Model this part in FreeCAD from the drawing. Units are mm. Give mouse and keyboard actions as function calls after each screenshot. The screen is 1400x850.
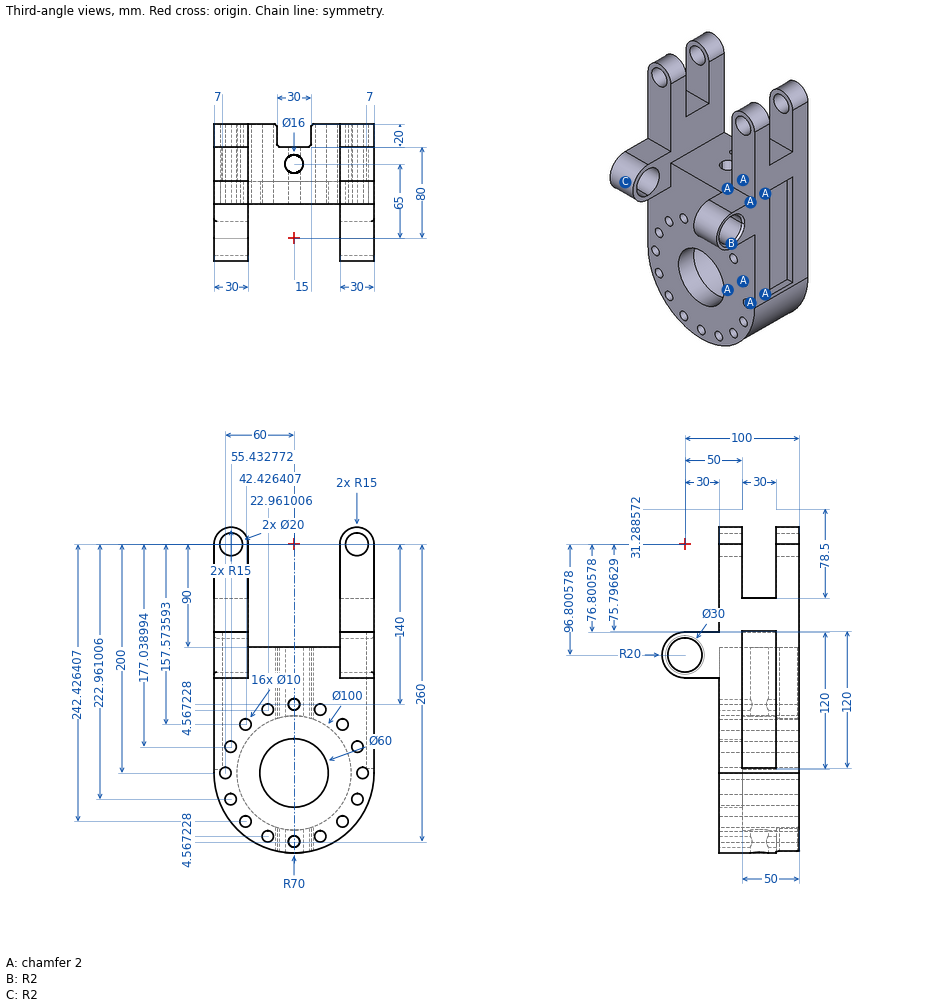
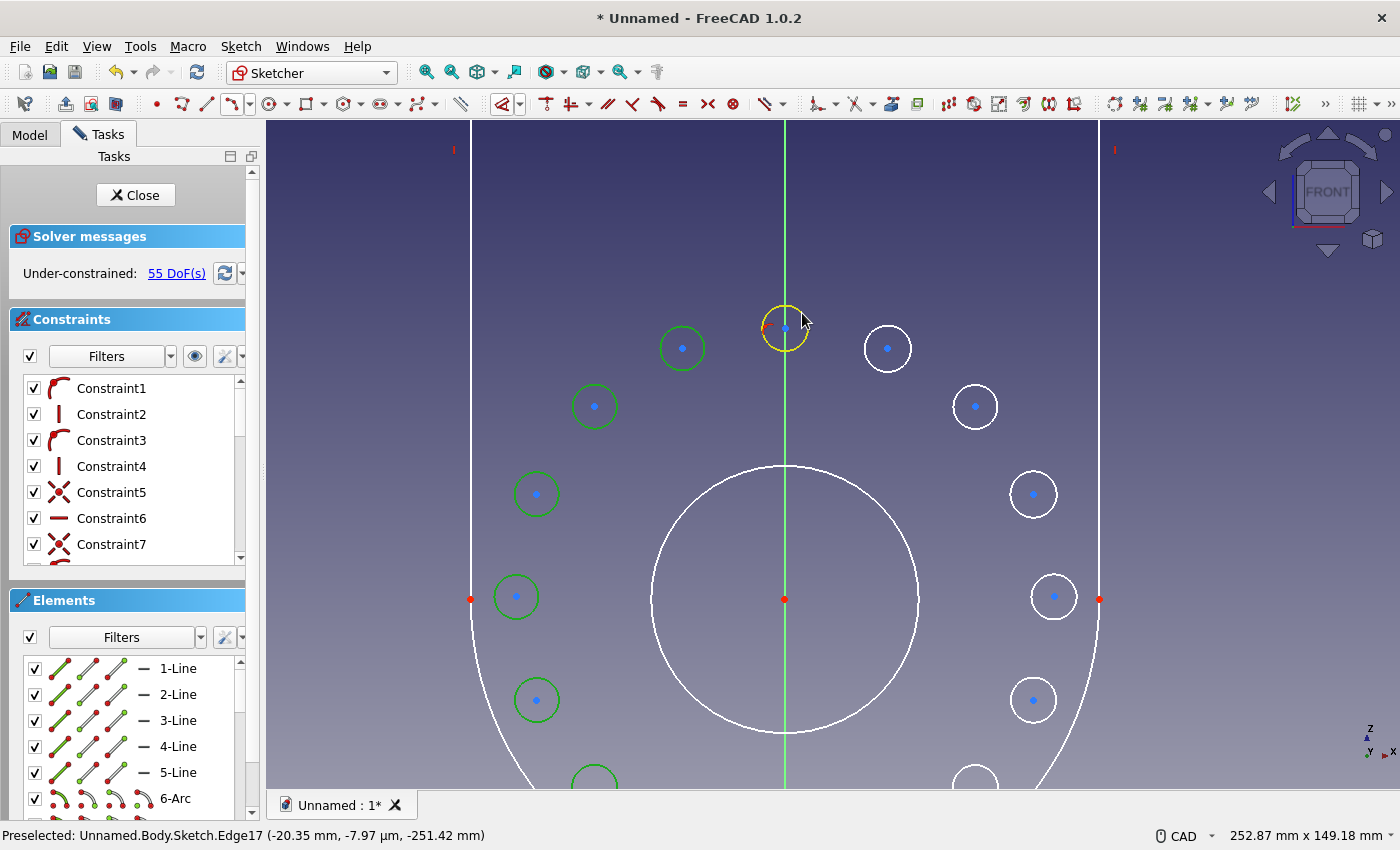
click(801, 312)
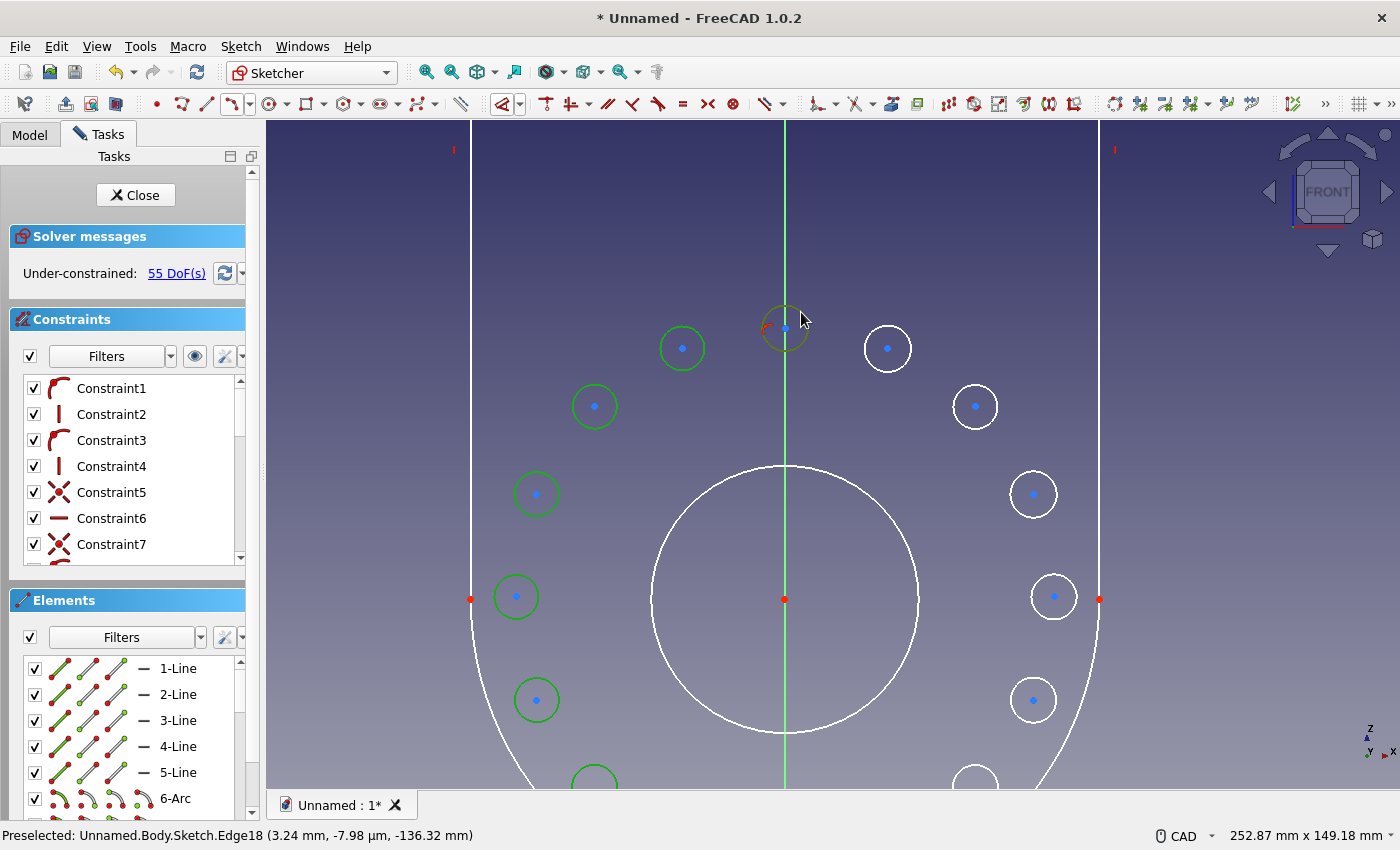
click(904, 332)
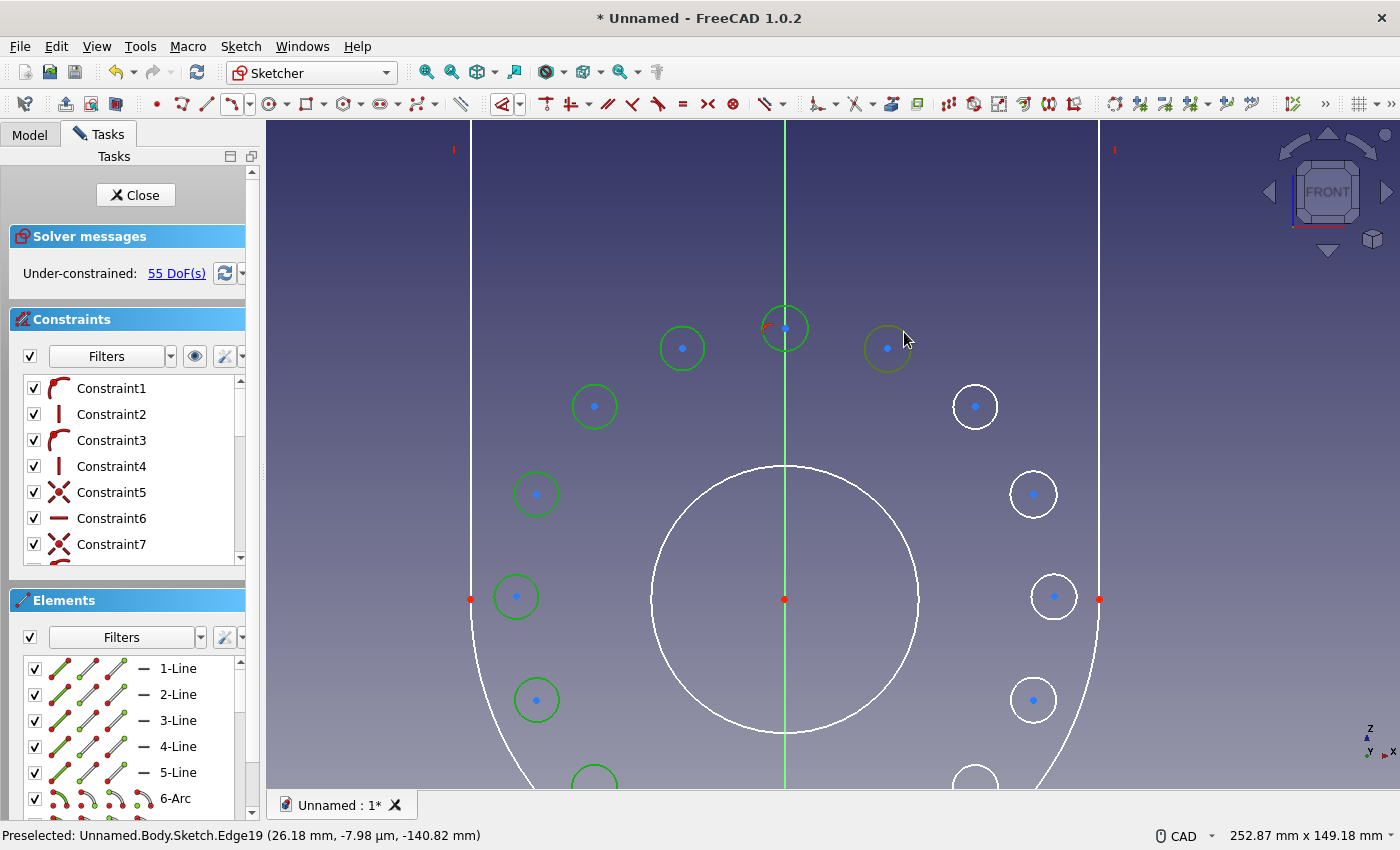
click(991, 391)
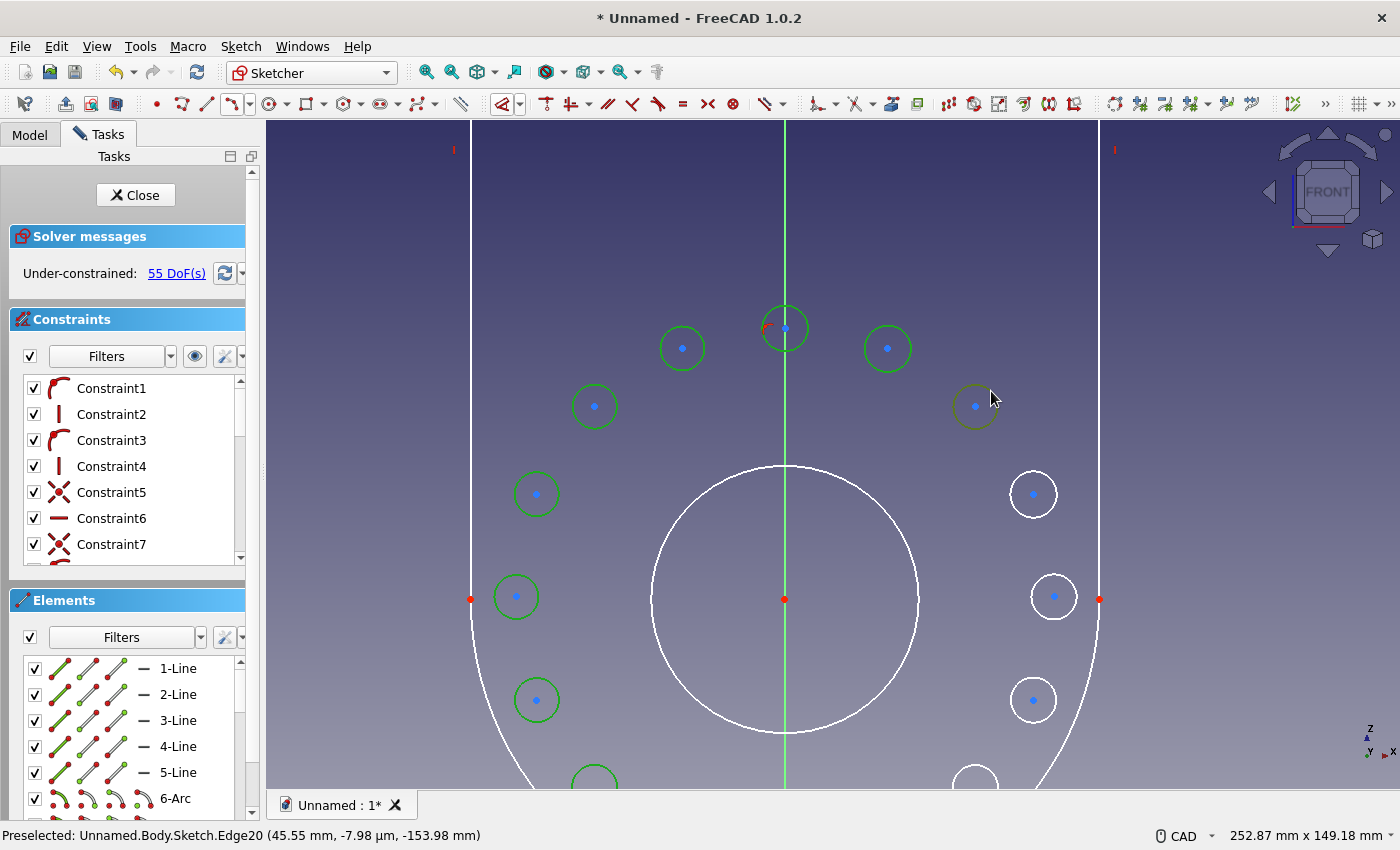
click(1050, 478)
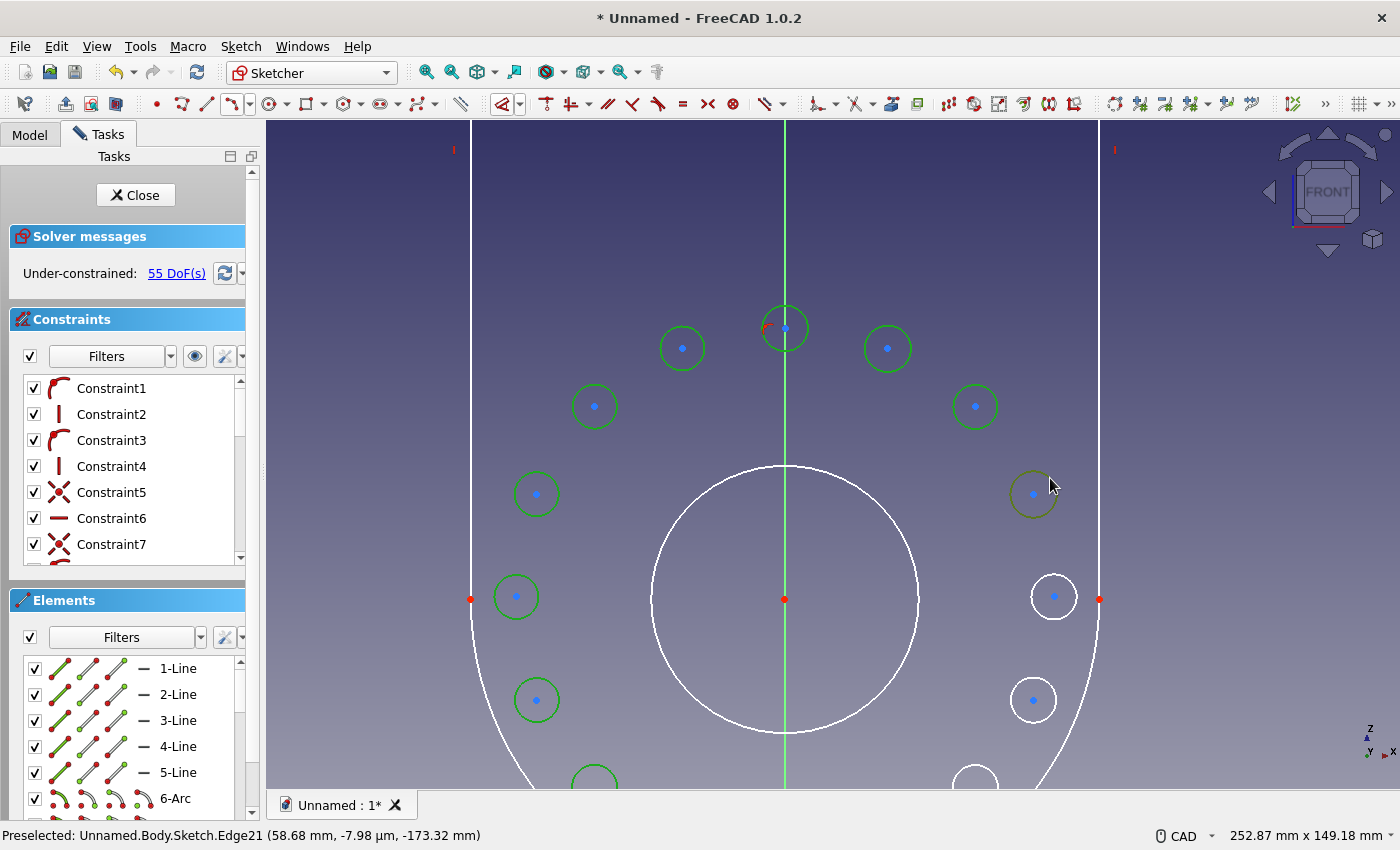
scroll(752, 561, down, 5)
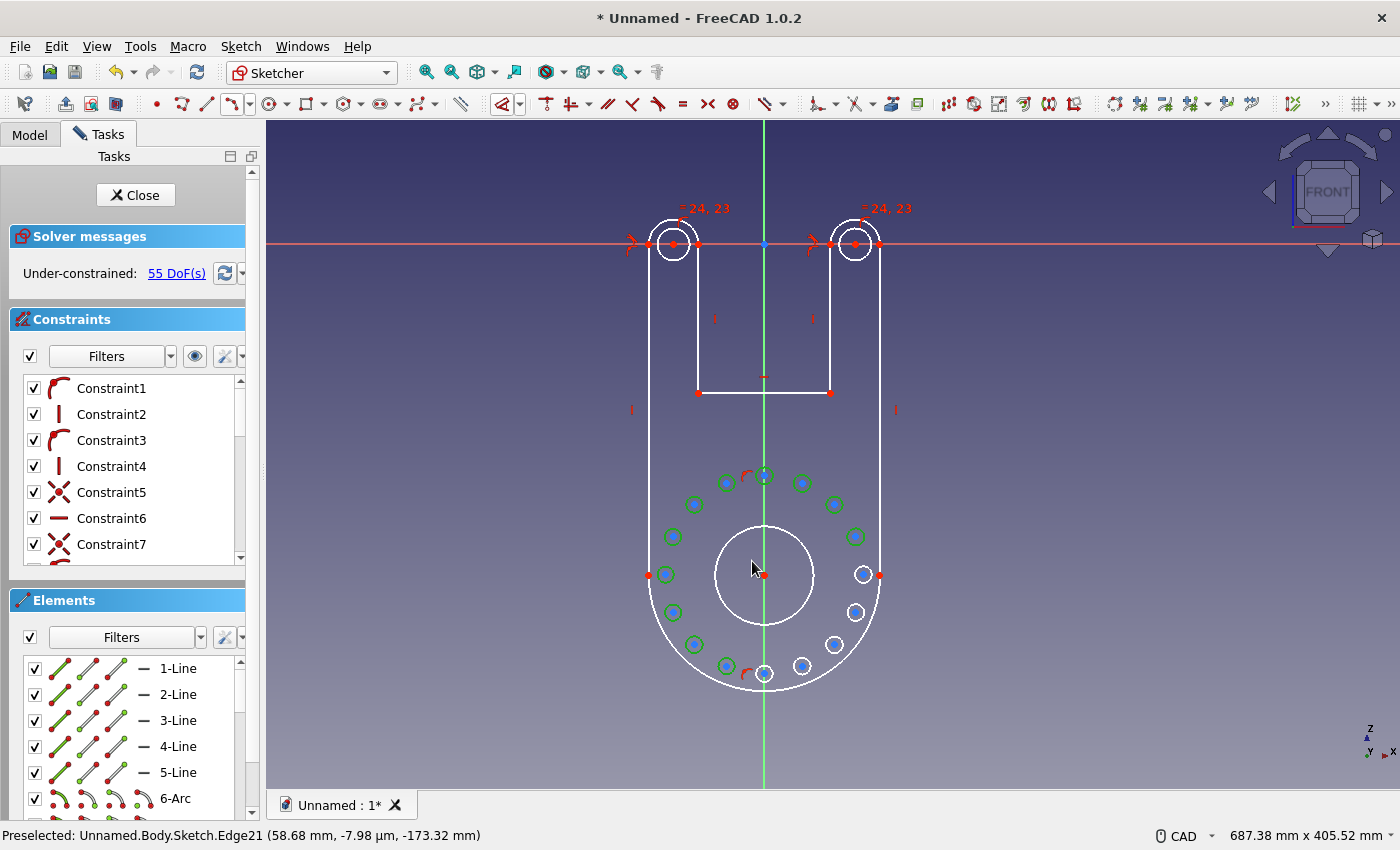
scroll(770, 668, up, 5)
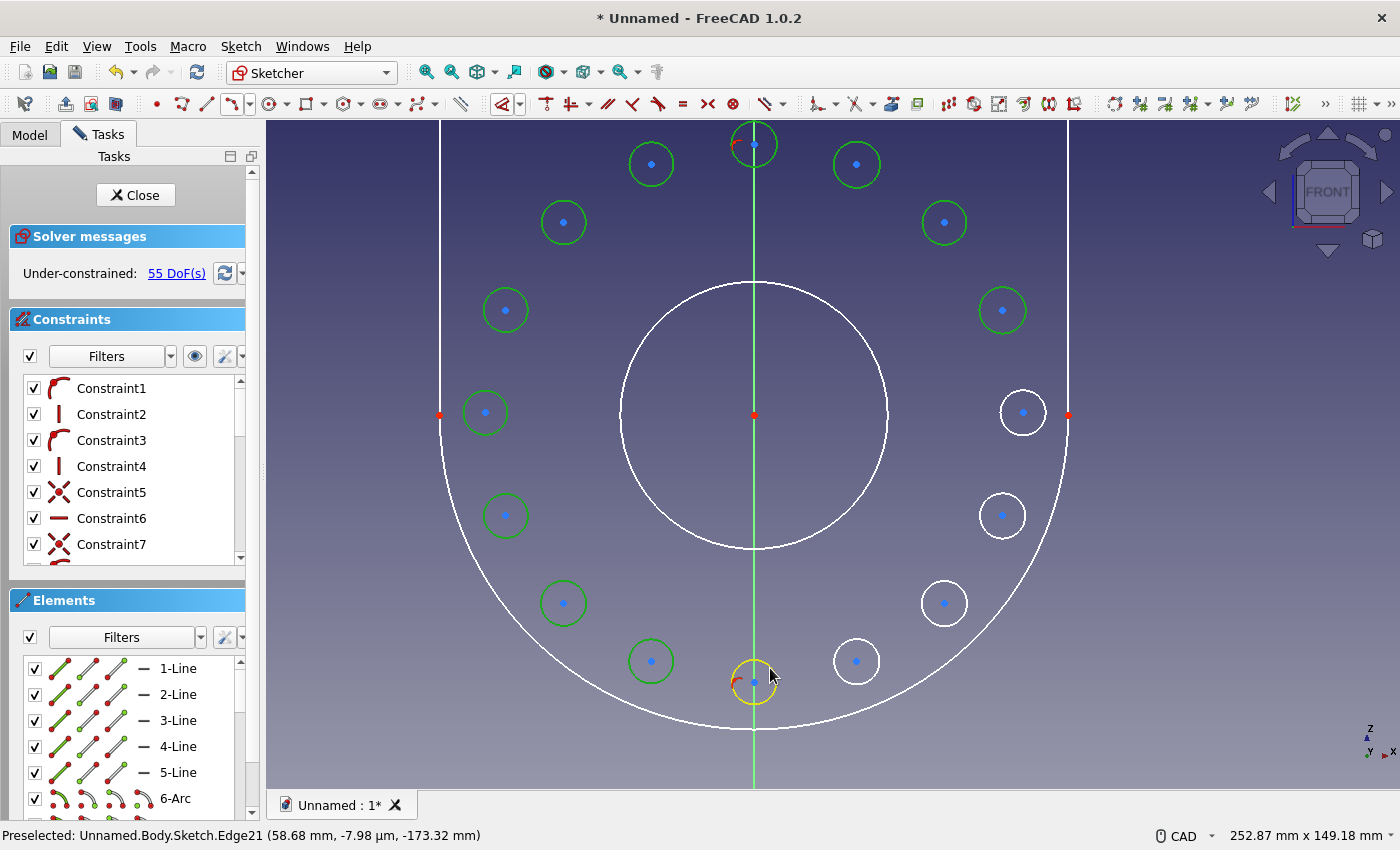
click(770, 666)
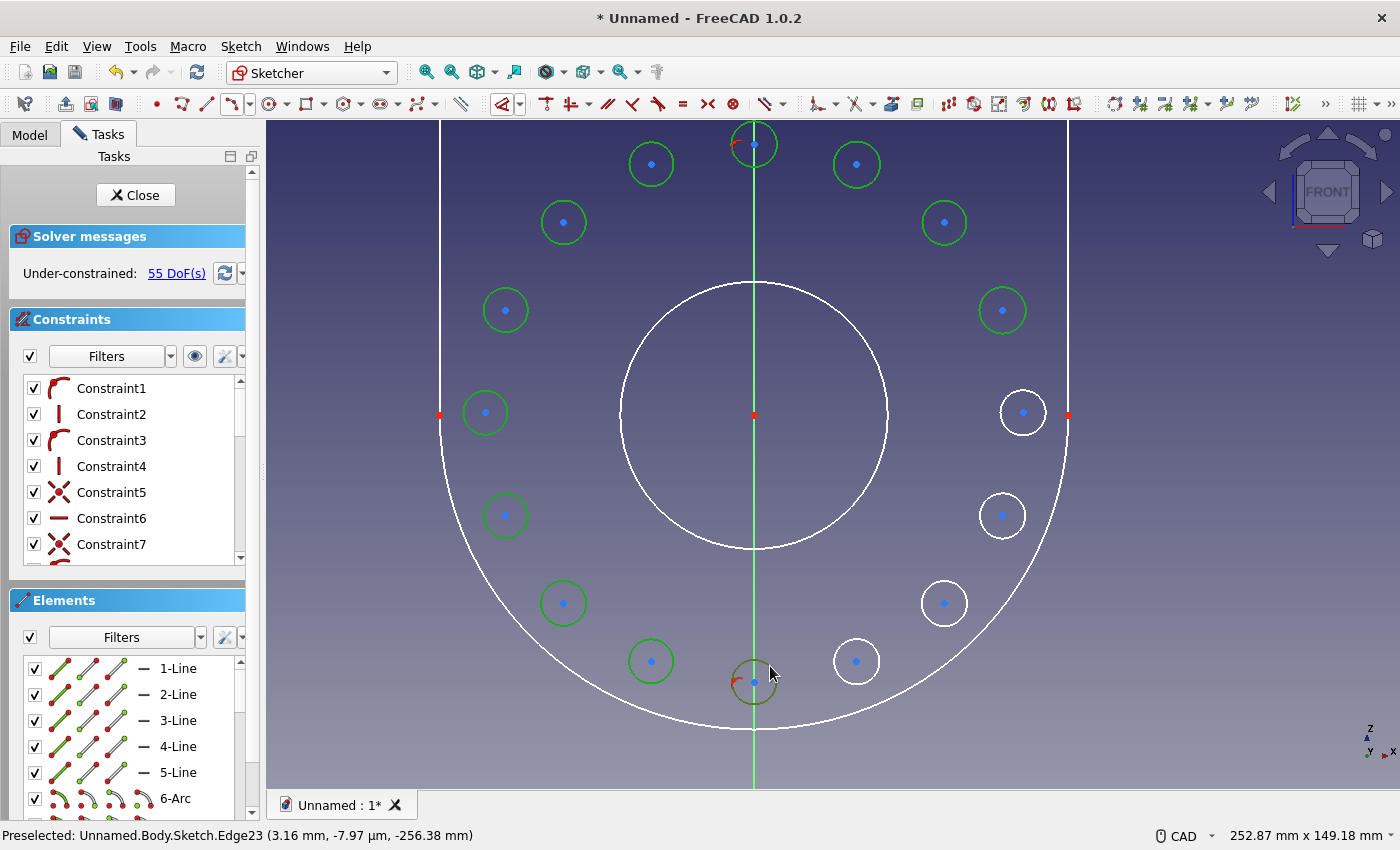
click(873, 646)